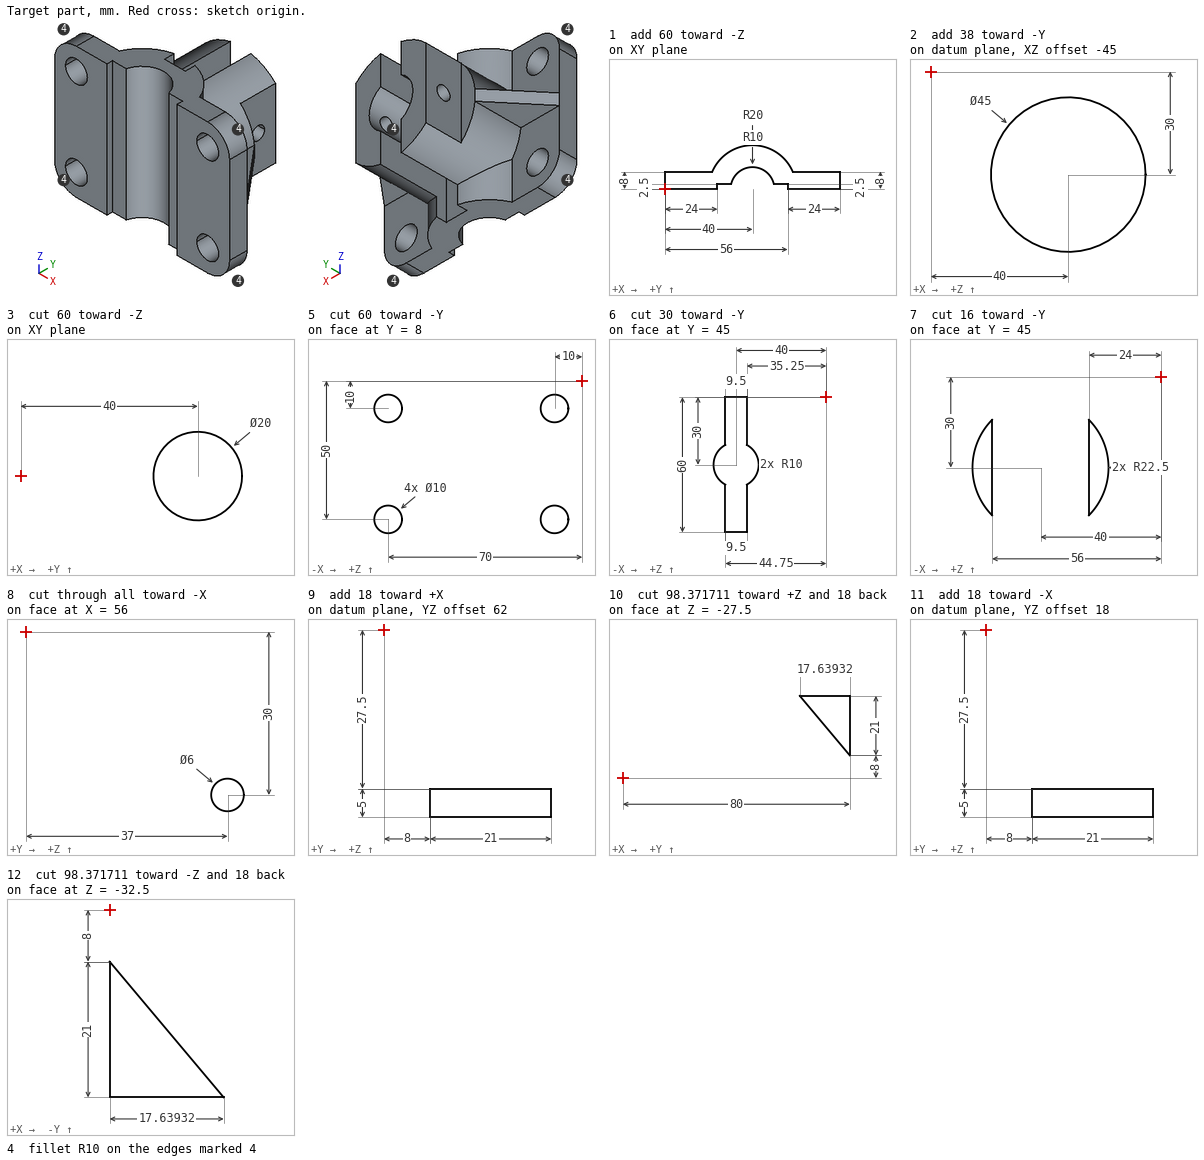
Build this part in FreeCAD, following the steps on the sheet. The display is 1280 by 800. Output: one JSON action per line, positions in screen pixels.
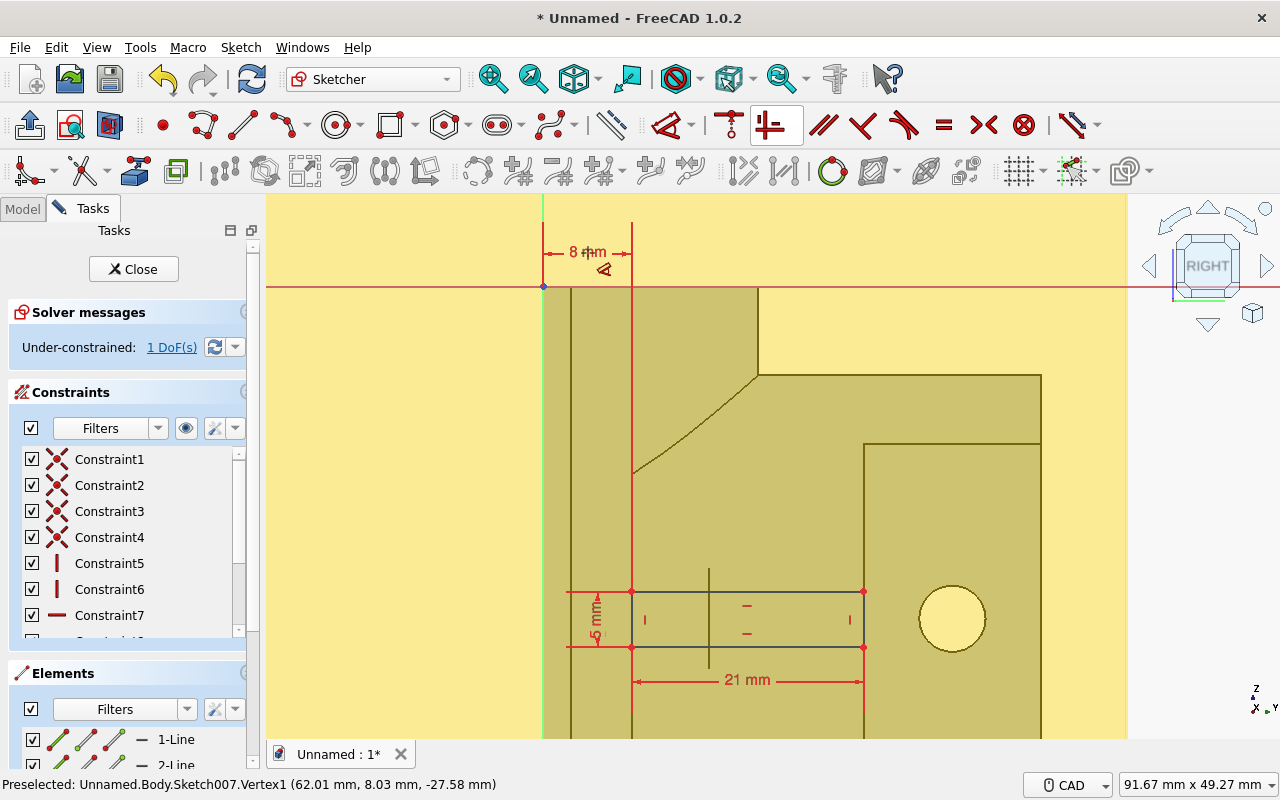
{"action": "left_click", "coordinate": [632, 592]}
{"action": "left_click", "coordinate": [509, 439]}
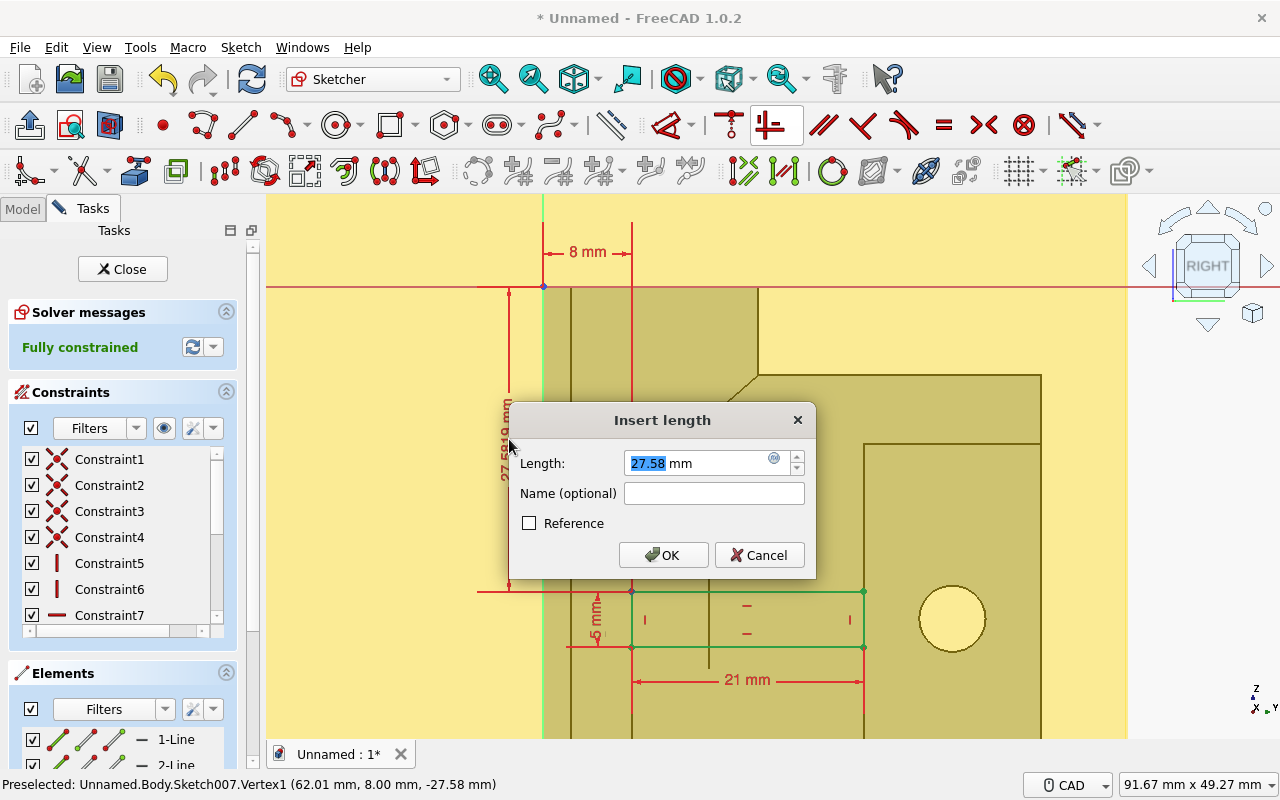
{"action": "type", "text": "27.5"}
{"action": "key", "text": "Return"}
{"action": "key", "text": "Escape"}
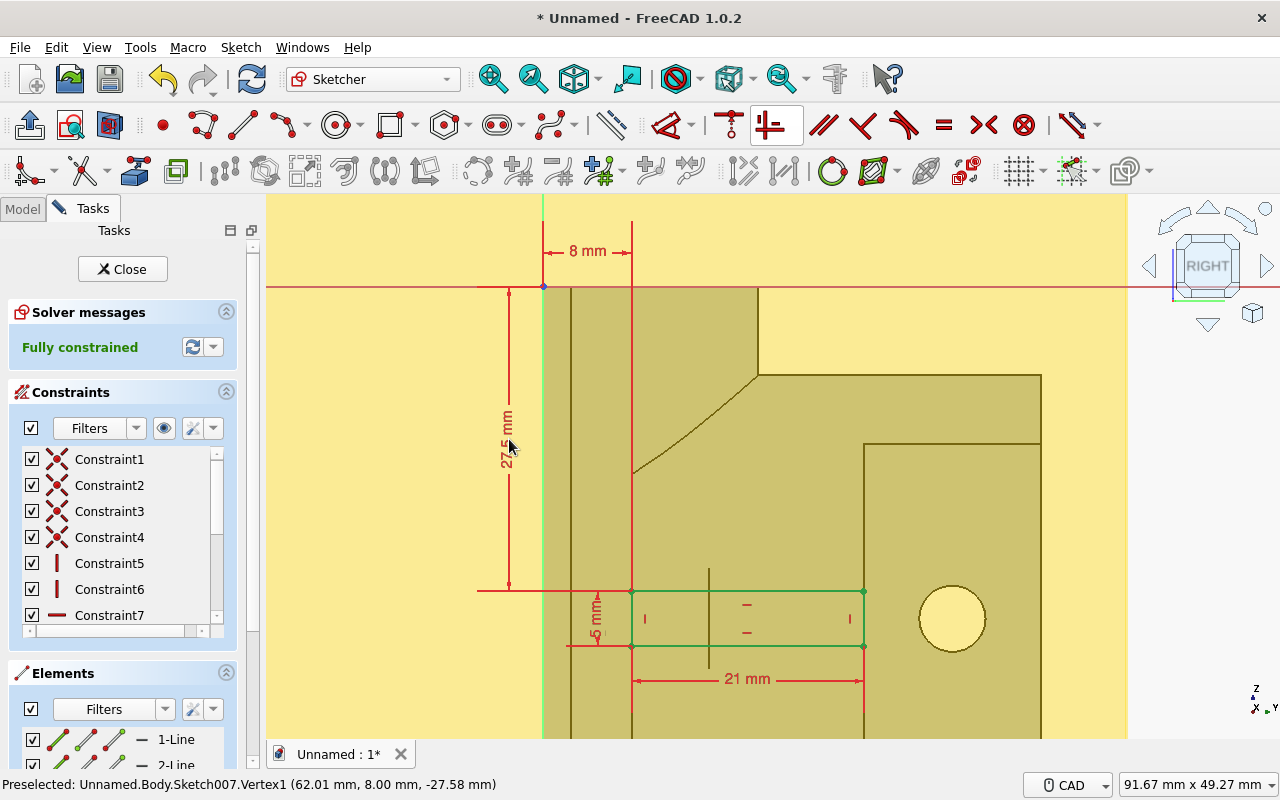
{"action": "left_click", "coordinate": [123, 269]}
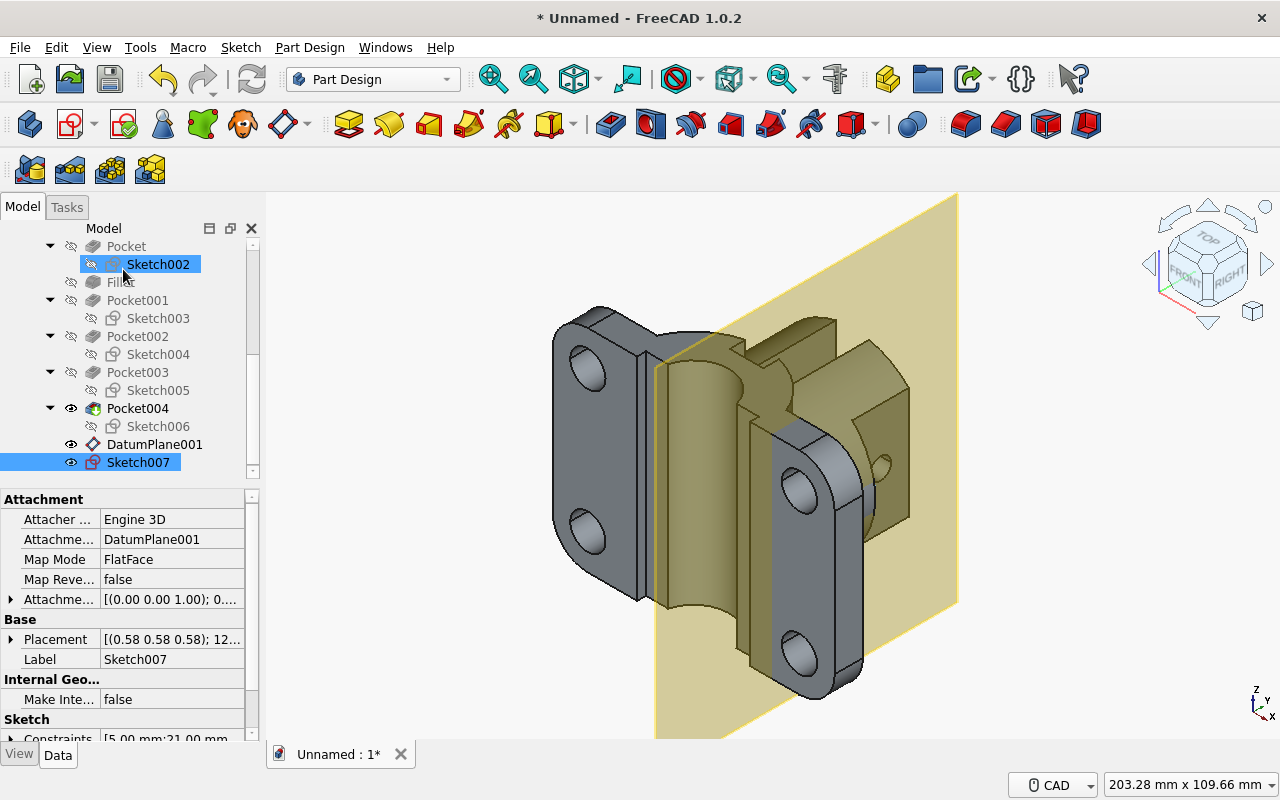
{"action": "left_click", "coordinate": [350, 124]}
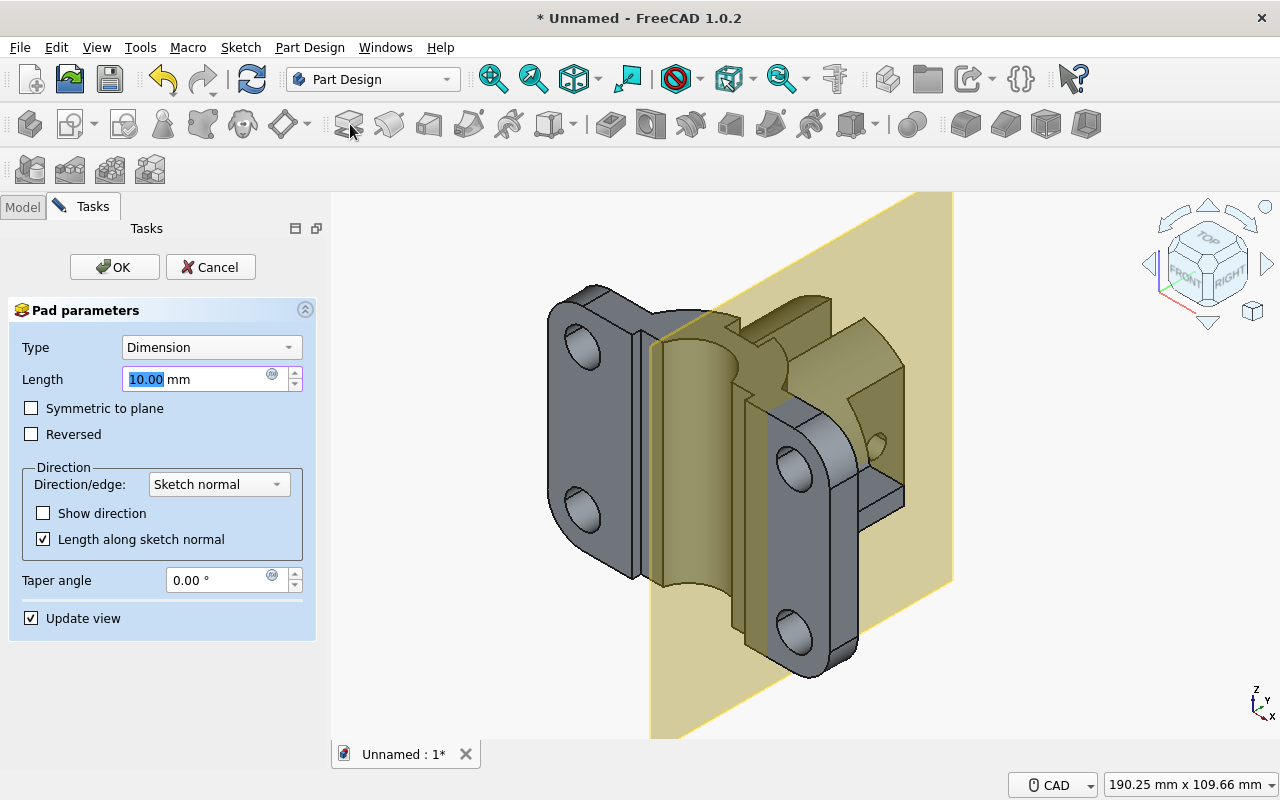
{"action": "type", "text": "18"}
{"action": "key", "text": "Tab"}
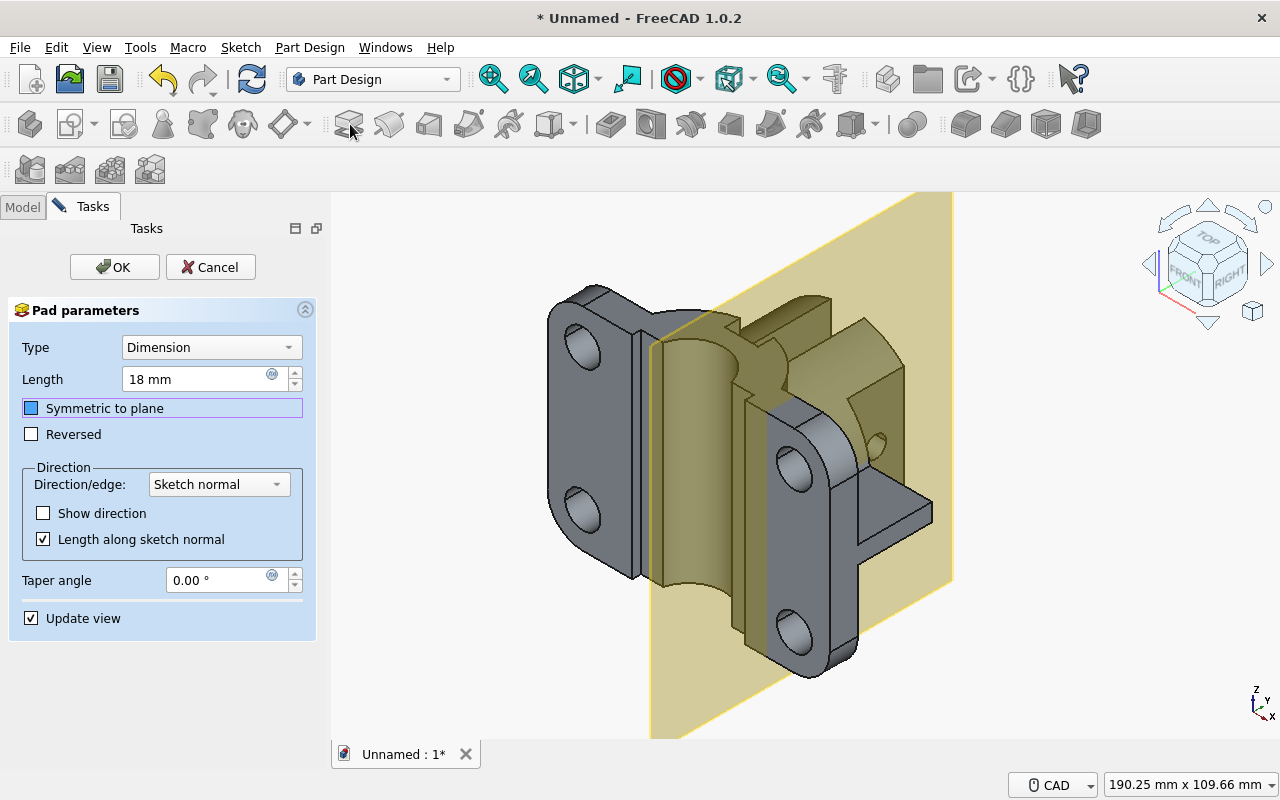
{"action": "left_click", "coordinate": [115, 267]}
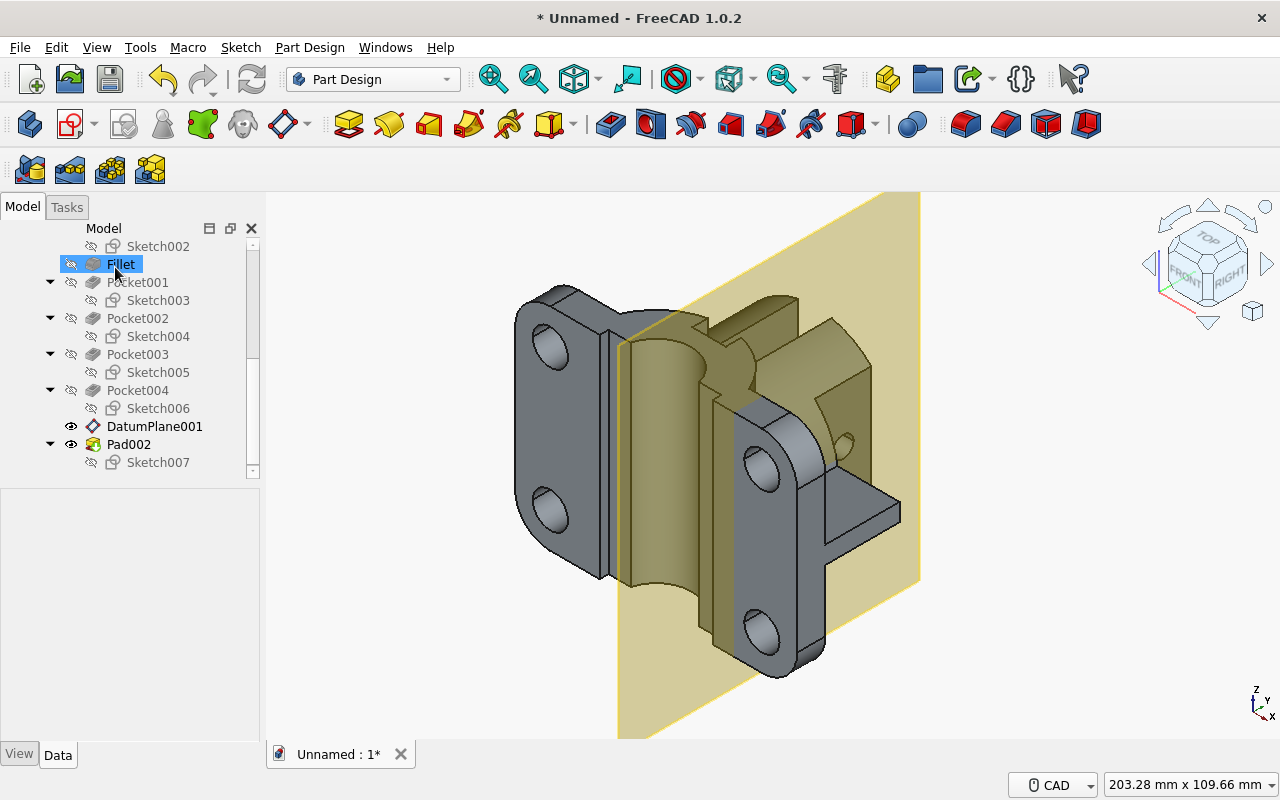
{"action": "left_click", "coordinate": [116, 426]}
{"action": "key", "text": "space"}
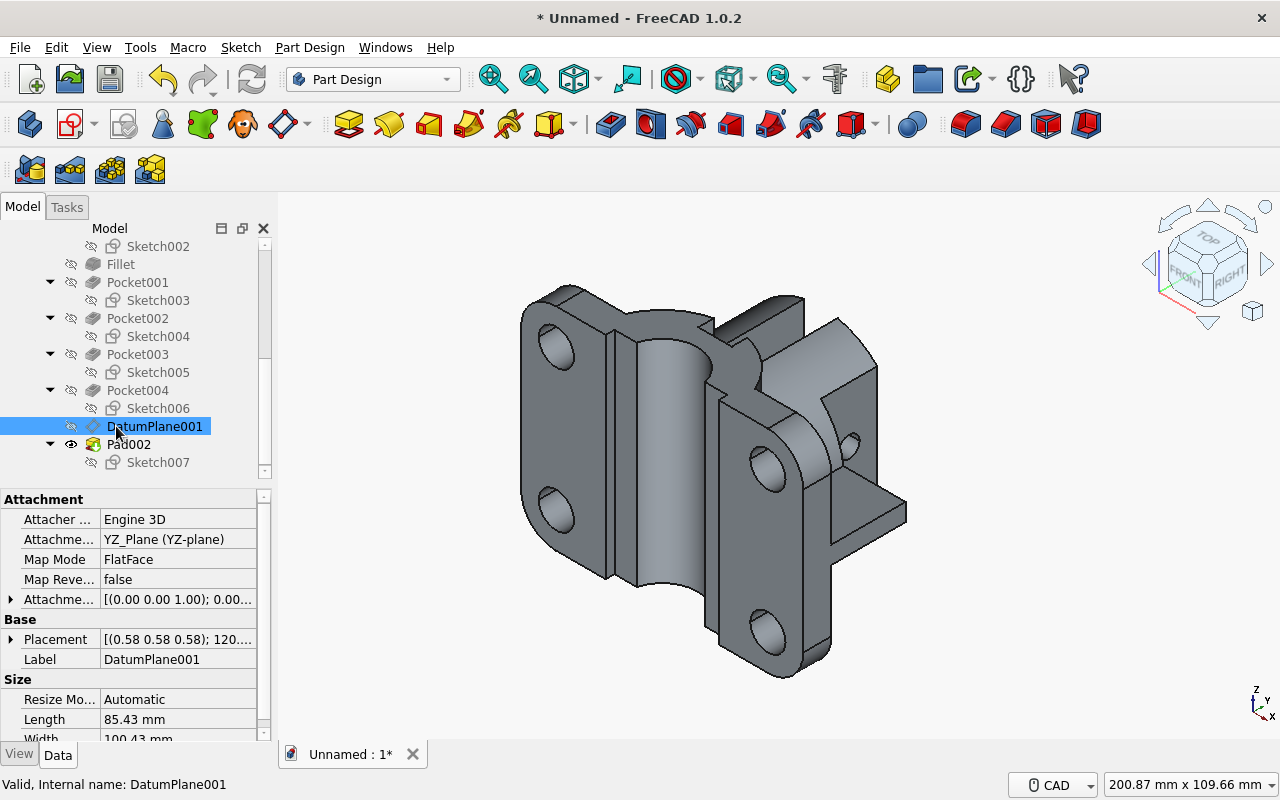
{"action": "left_click", "coordinate": [848, 498]}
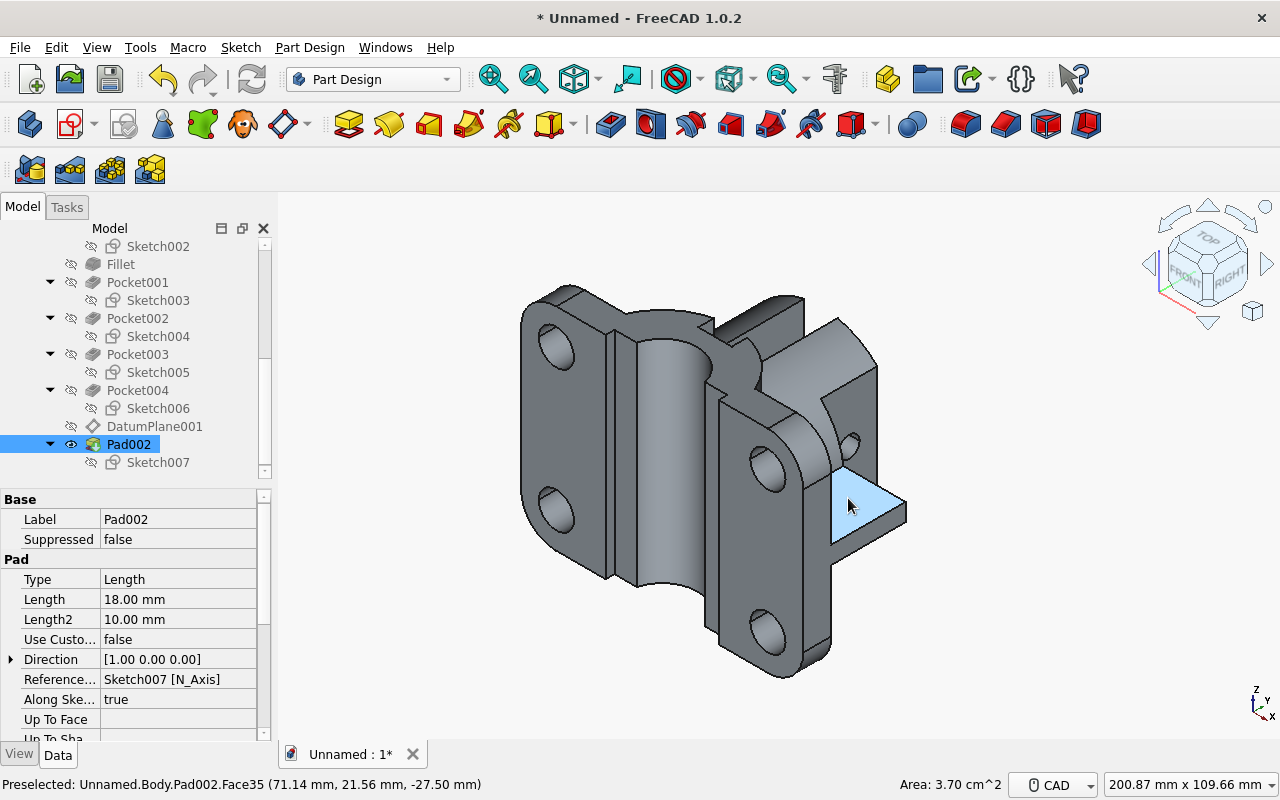
{"action": "left_click", "coordinate": [70, 124]}